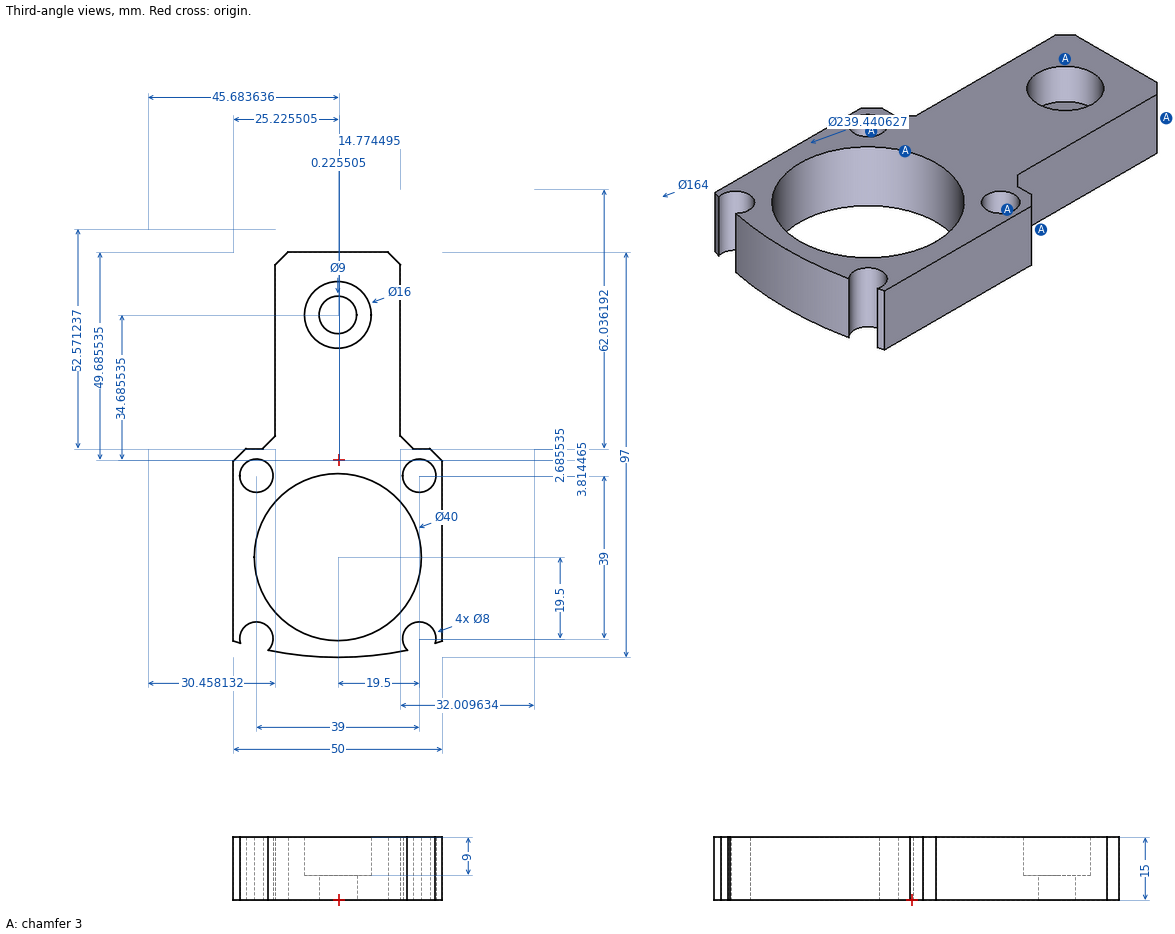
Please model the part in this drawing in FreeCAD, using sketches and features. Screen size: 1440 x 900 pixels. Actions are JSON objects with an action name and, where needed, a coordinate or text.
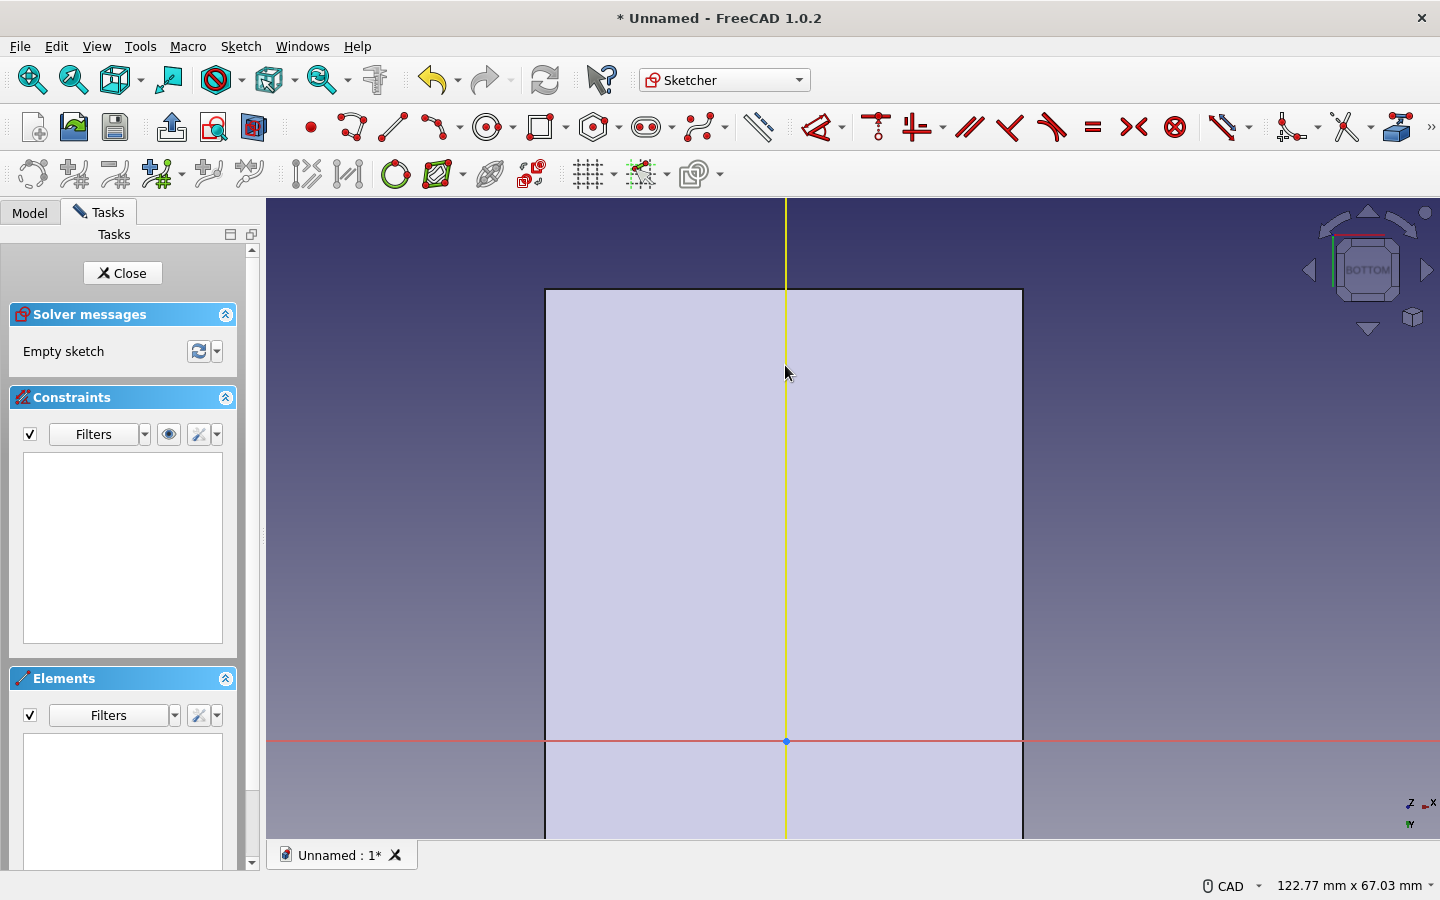
{"action": "left_click", "coordinate": [486, 128]}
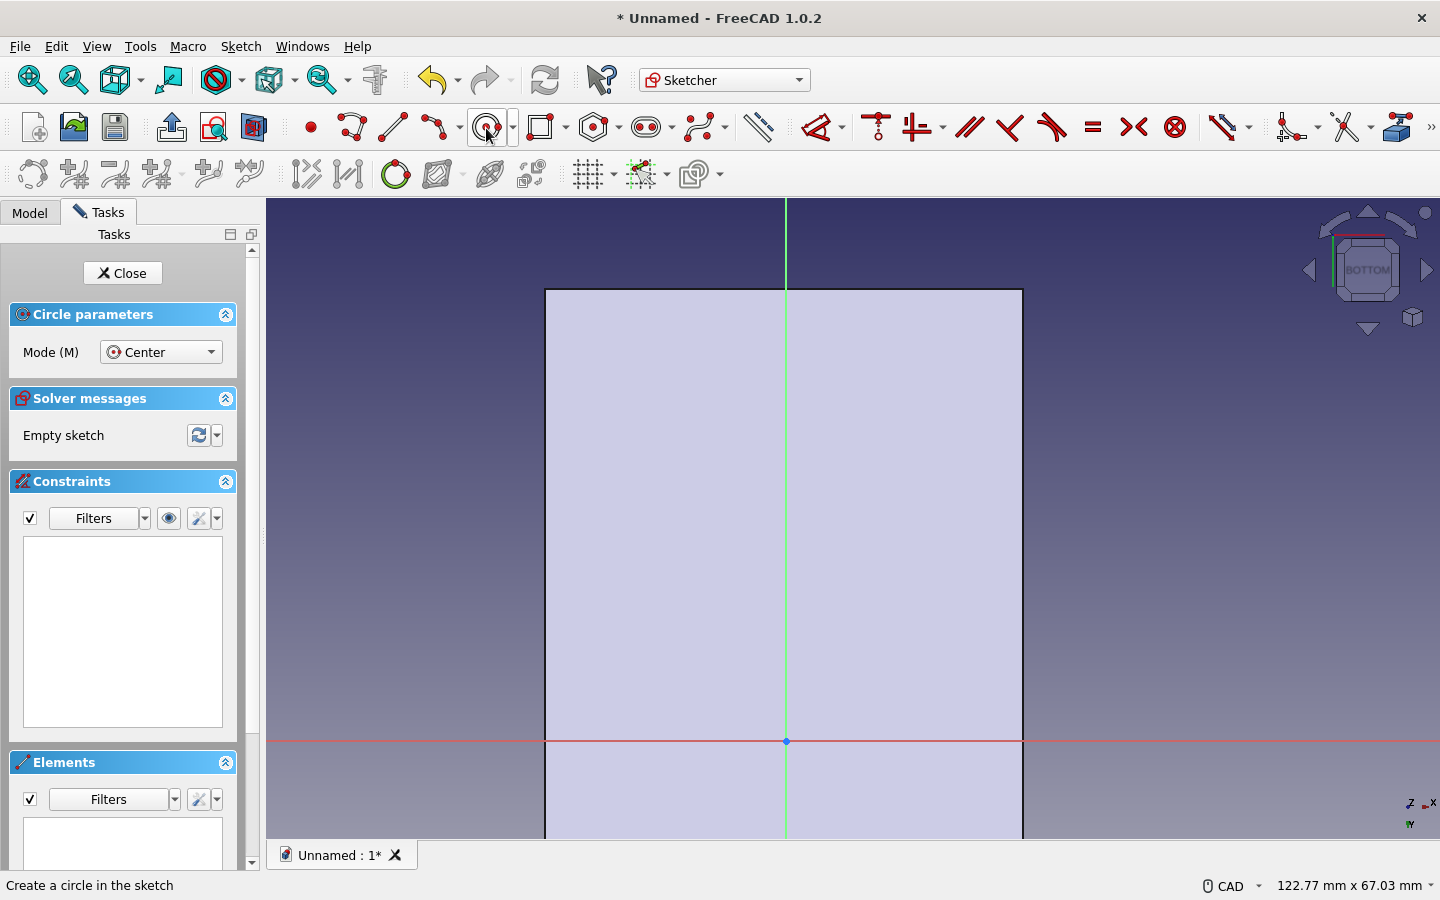
{"action": "scroll", "coordinate": [784, 518], "scroll_direction": "up", "scroll_amount": 10}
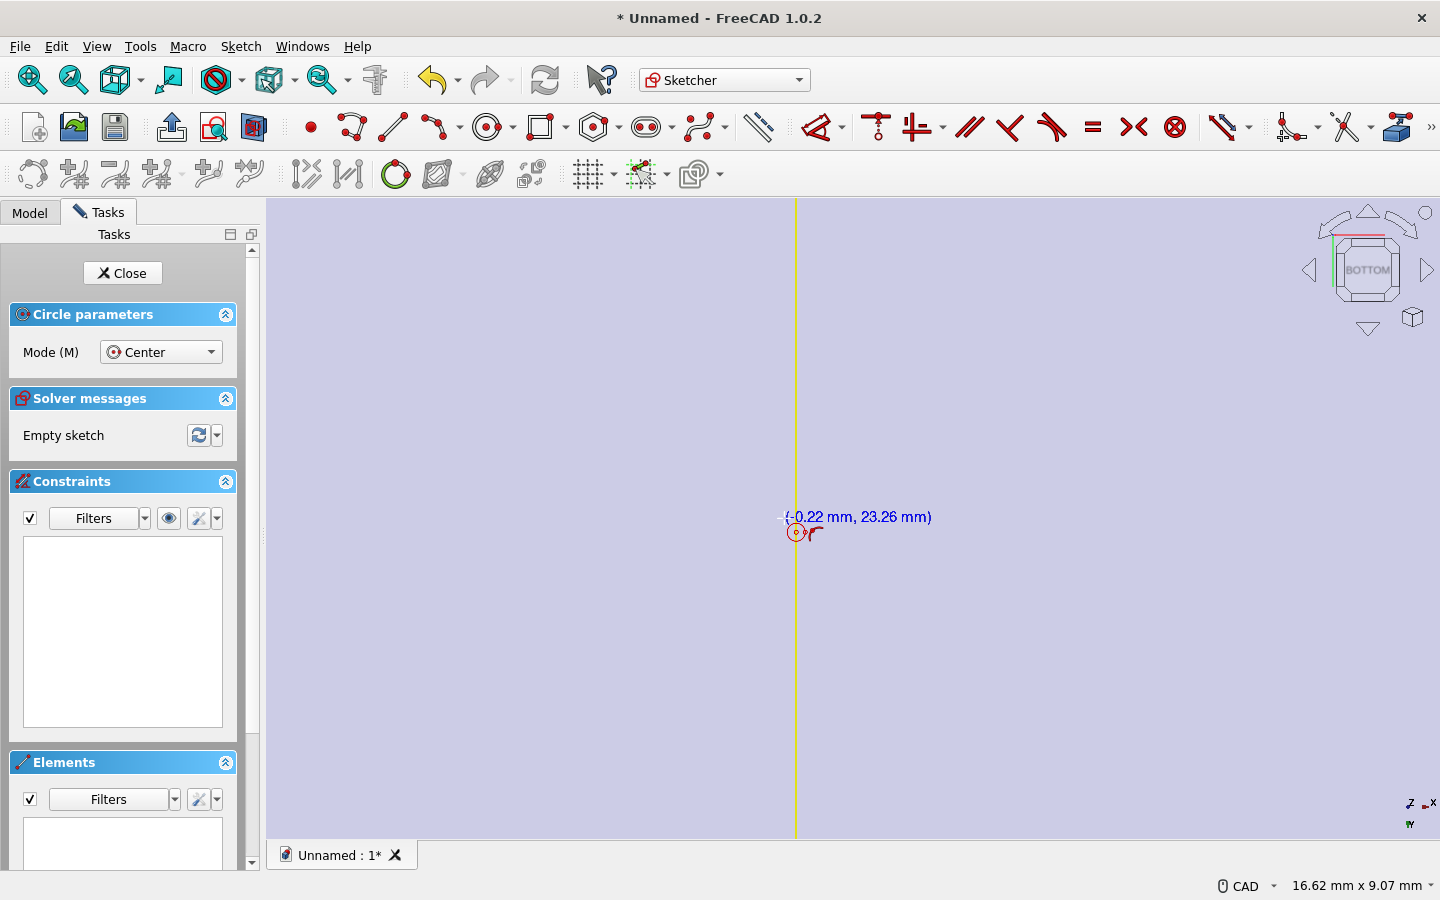
{"action": "left_click", "coordinate": [780, 518]}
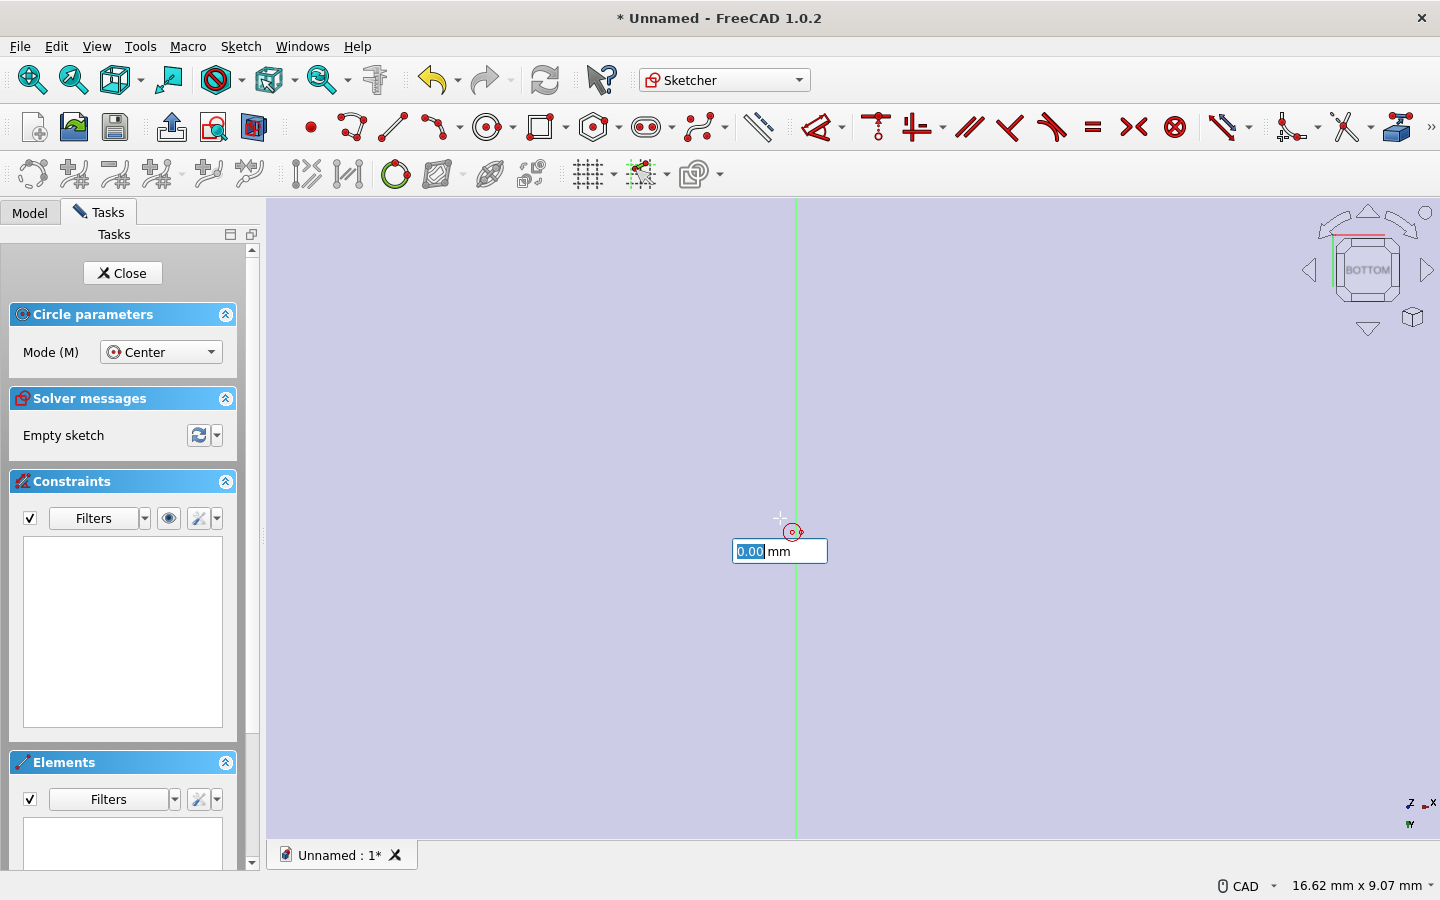
{"action": "scroll", "coordinate": [785, 519], "scroll_direction": "down", "scroll_amount": 10}
{"action": "mouse_move", "coordinate": [920, 384]}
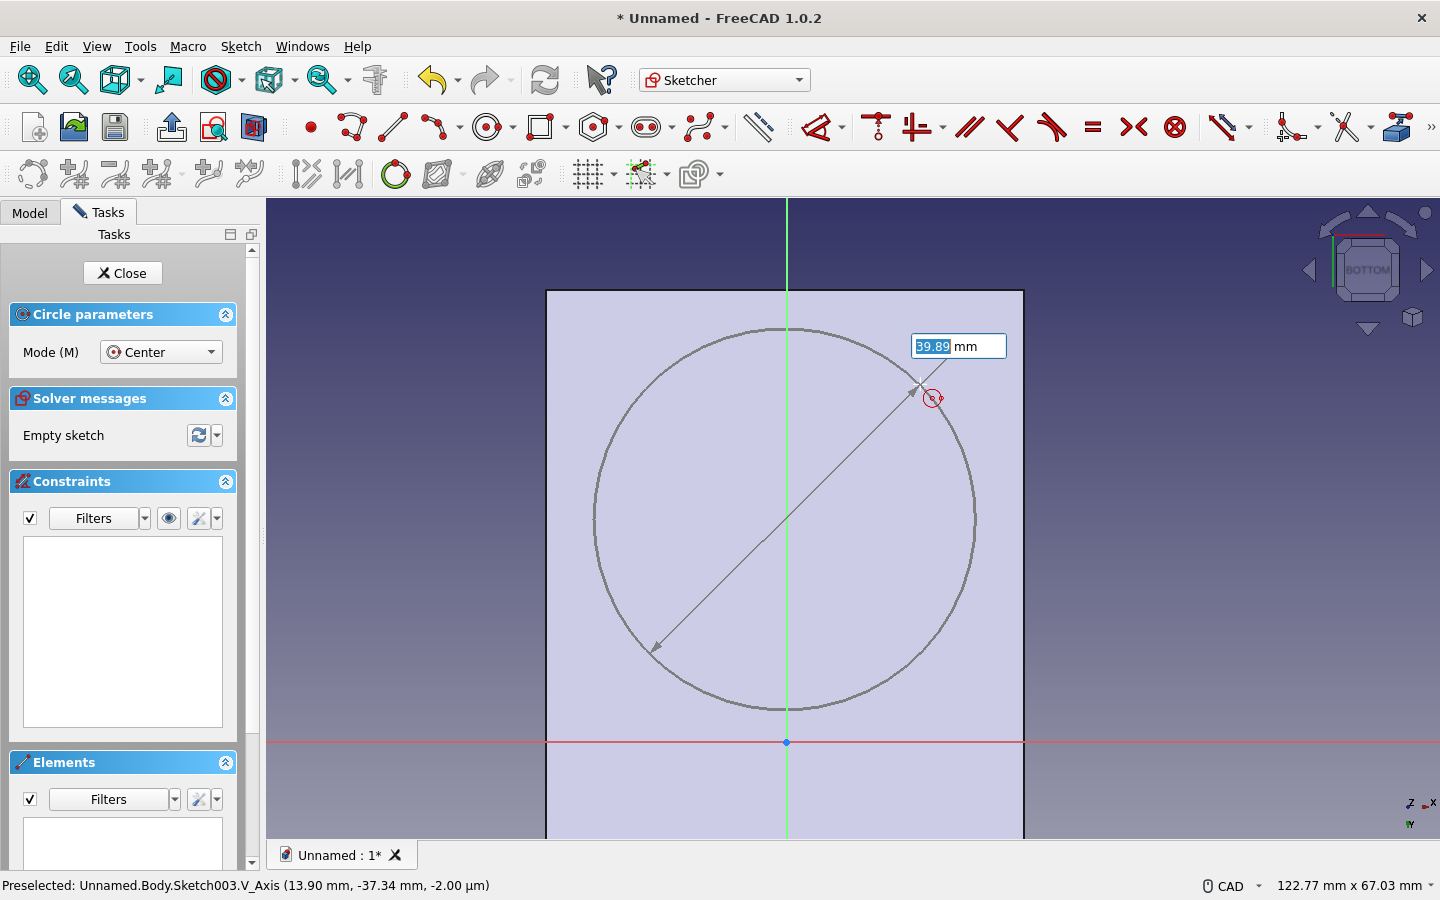
{"action": "type", "text": "40"}
{"action": "key", "text": "Return"}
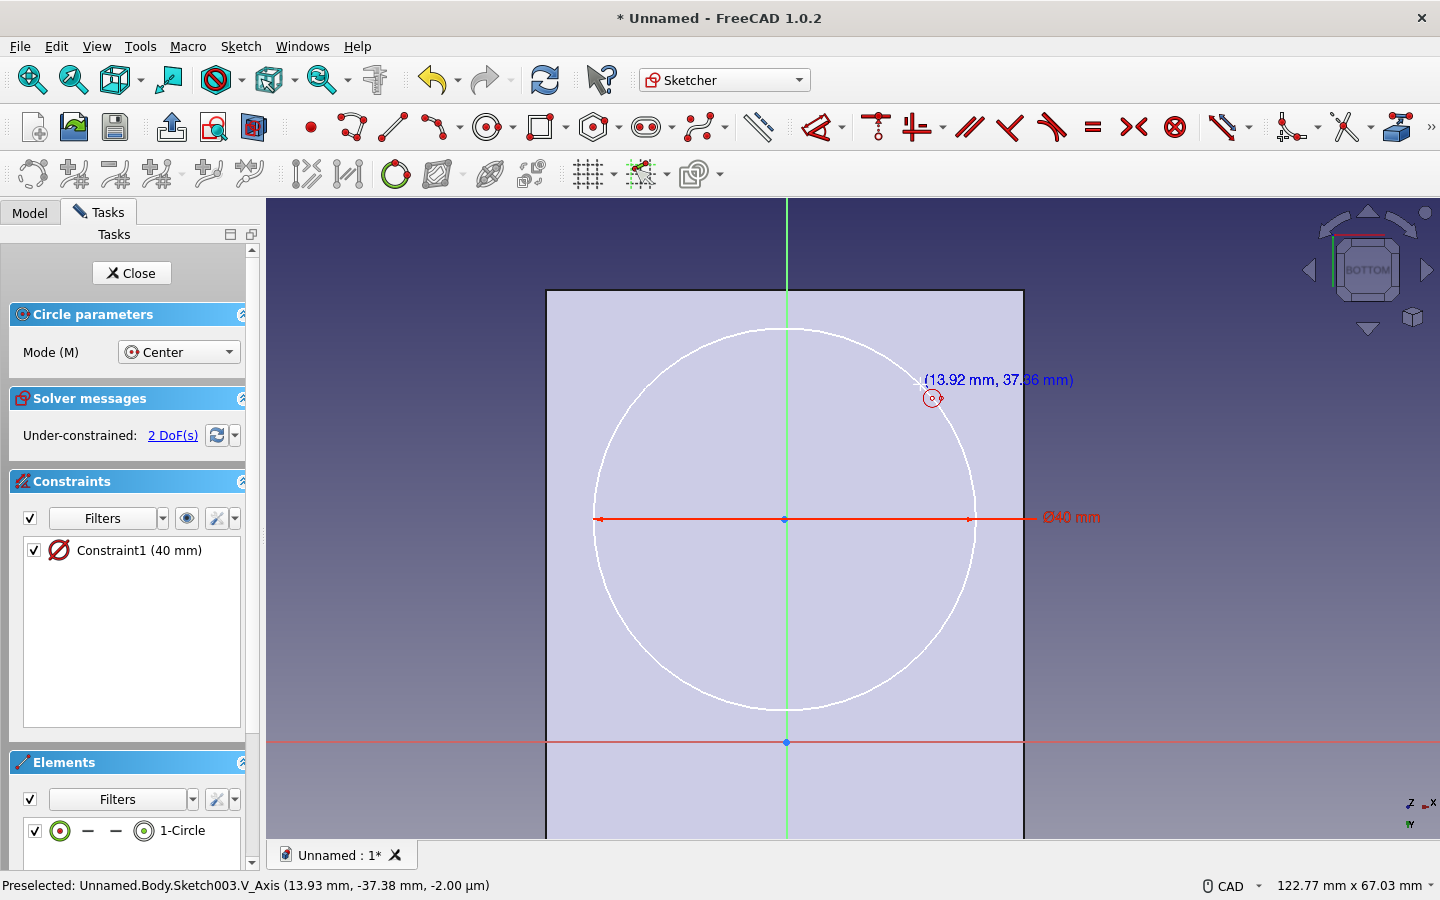
{"action": "left_click", "coordinate": [971, 333]}
{"action": "mouse_move", "coordinate": [998, 306]}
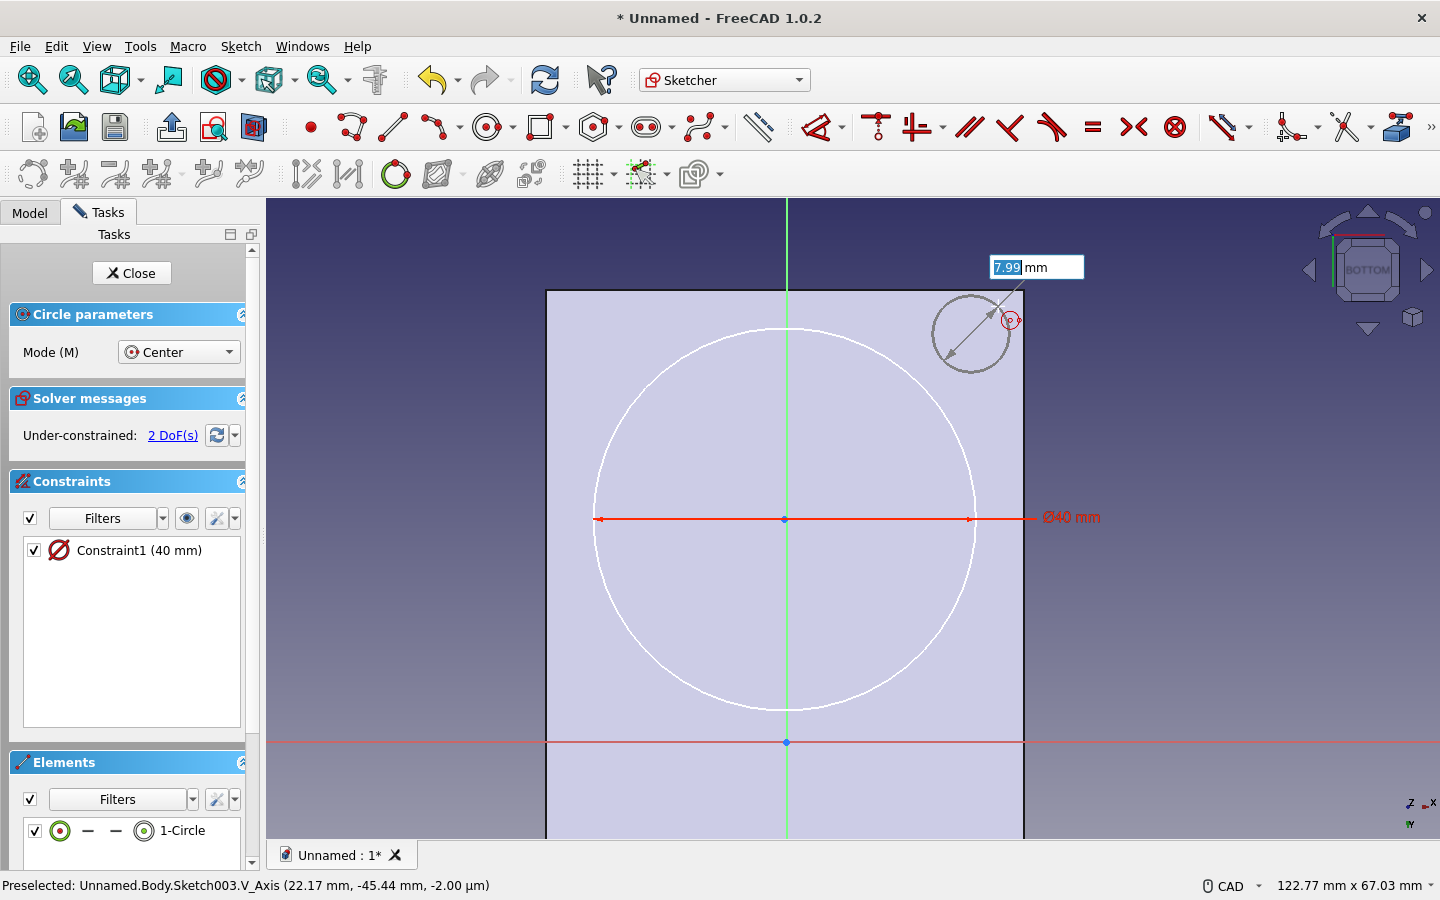
{"action": "type", "text": "8"}
{"action": "key", "text": "Return"}